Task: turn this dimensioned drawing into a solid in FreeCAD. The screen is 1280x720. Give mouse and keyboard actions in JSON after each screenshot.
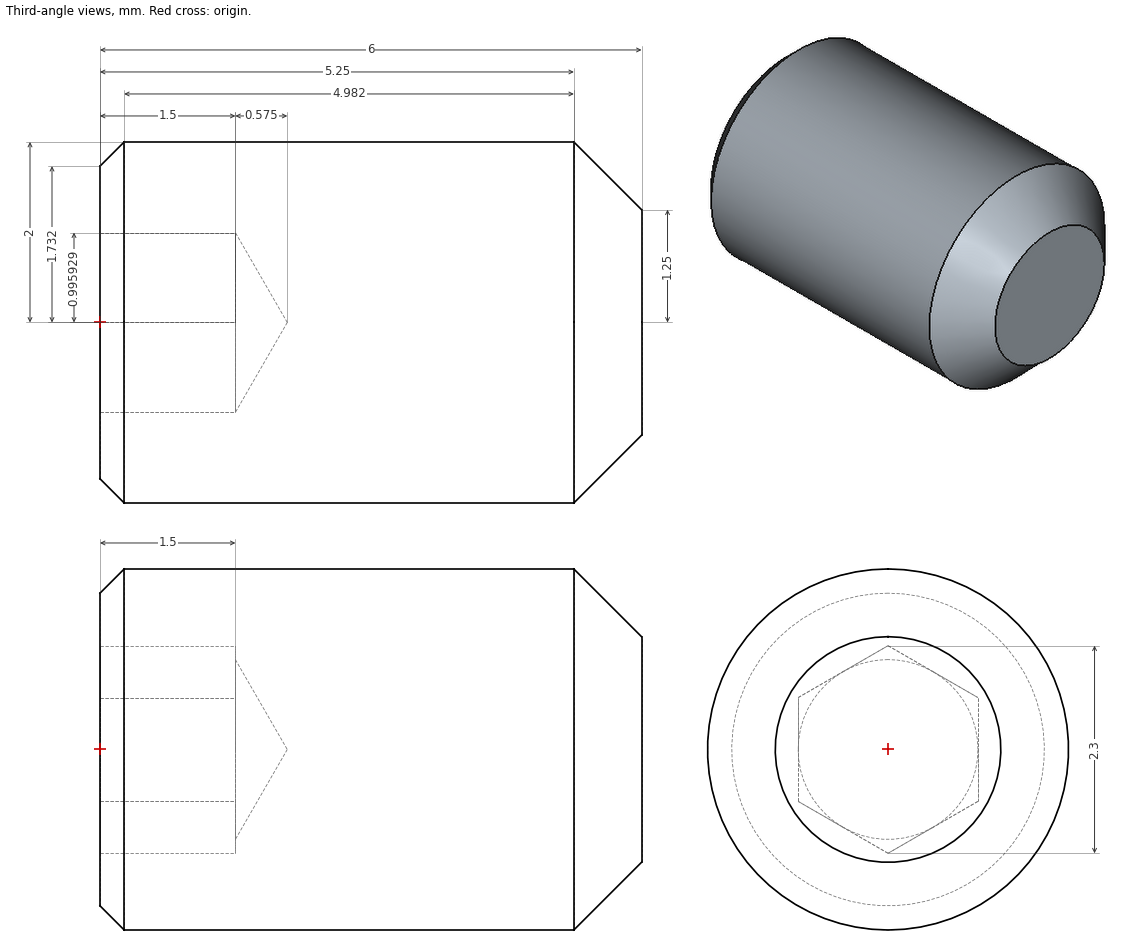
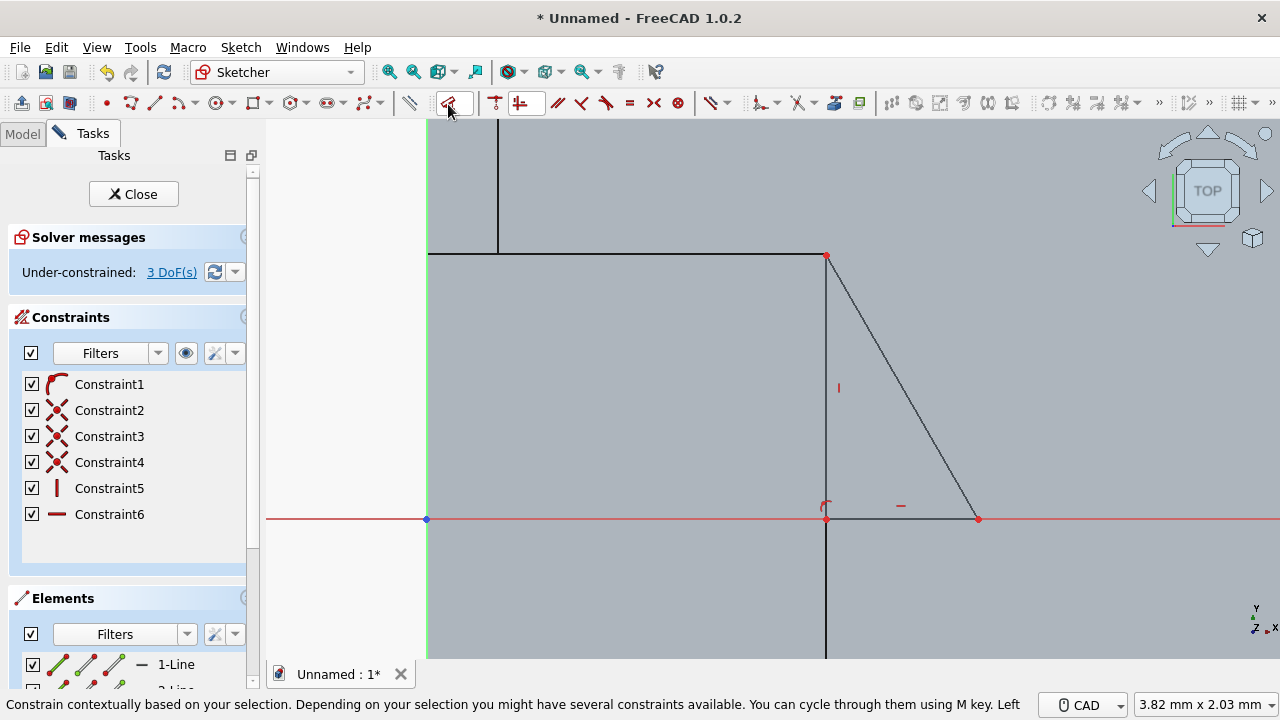
{"action": "left_click", "coordinate": [826, 519]}
{"action": "left_click", "coordinate": [626, 553]}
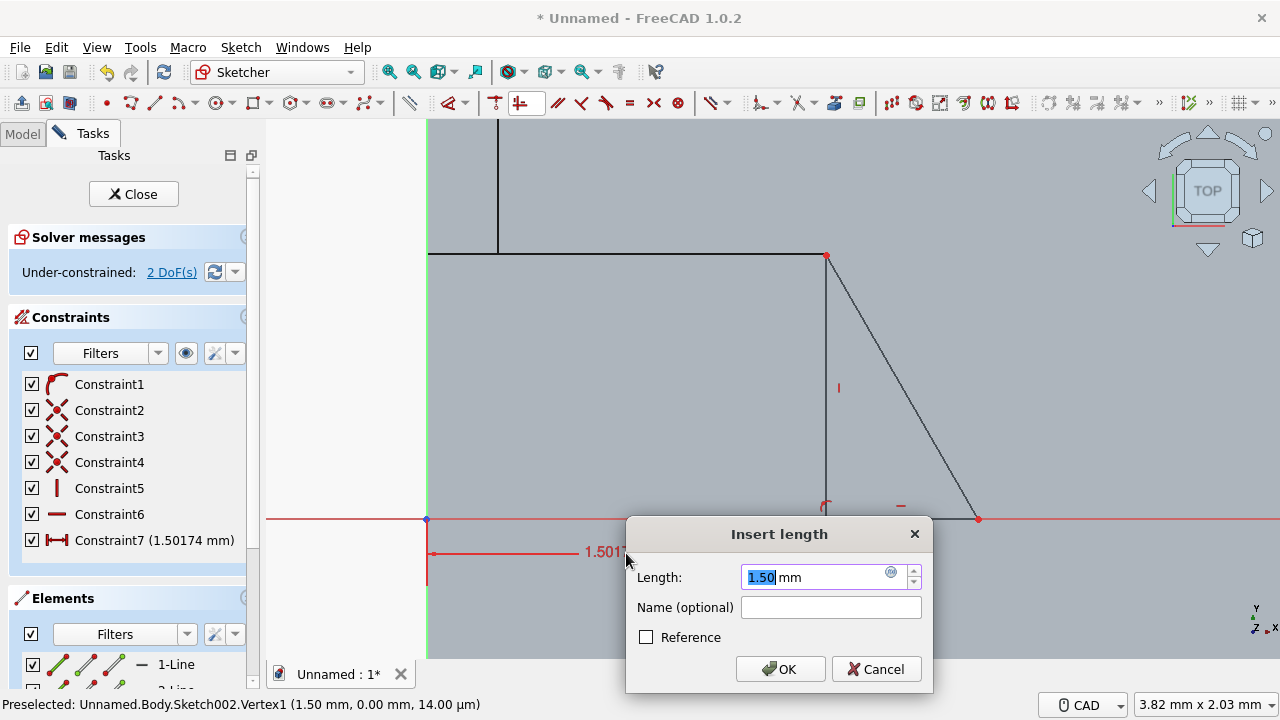
{"action": "type", "text": "1.5"}
{"action": "key", "text": "Return"}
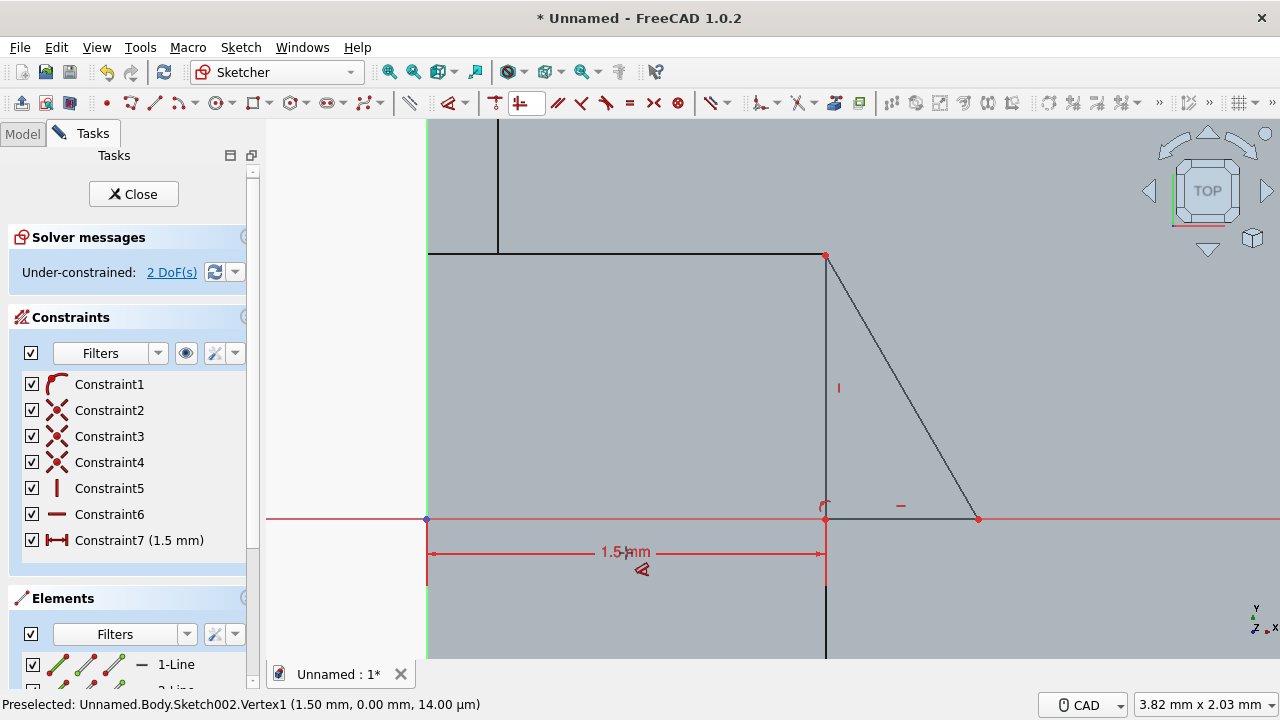
{"action": "left_click", "coordinate": [871, 519]}
{"action": "left_click", "coordinate": [902, 553]}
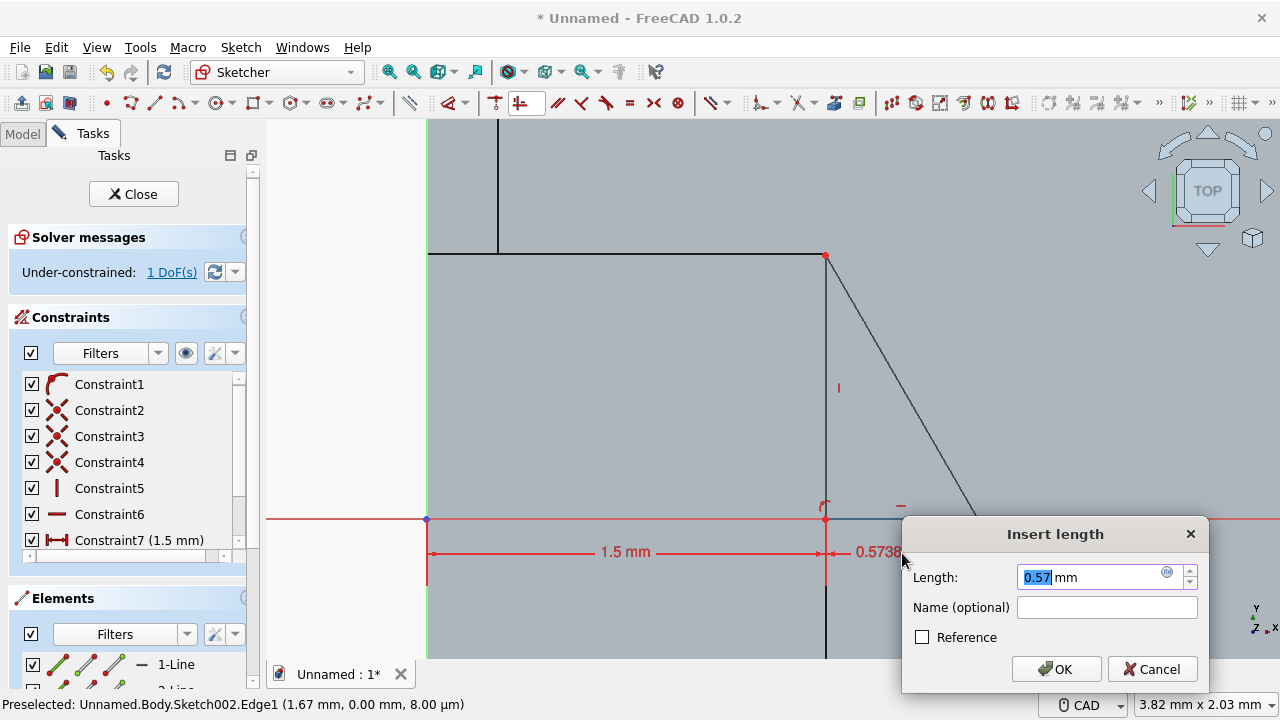
{"action": "type", "text": "0.575"}
{"action": "key", "text": "Return"}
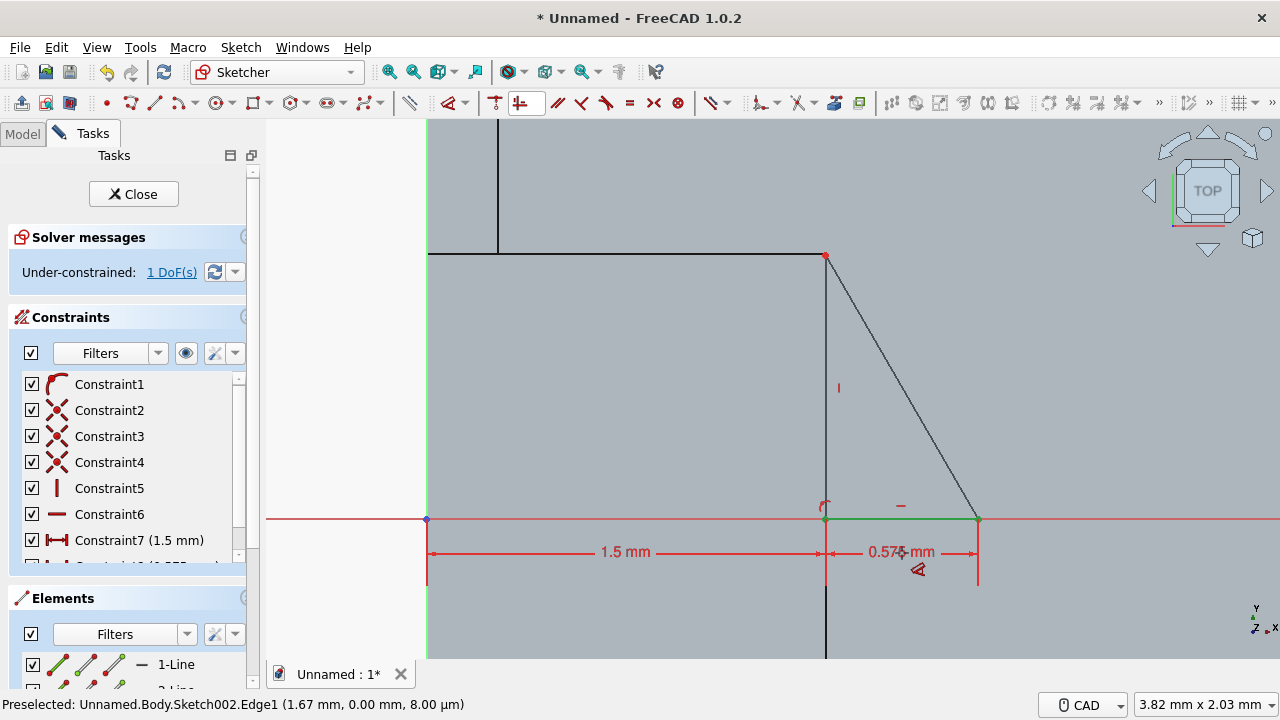
{"action": "left_click", "coordinate": [826, 334]}
{"action": "left_click", "coordinate": [860, 387]}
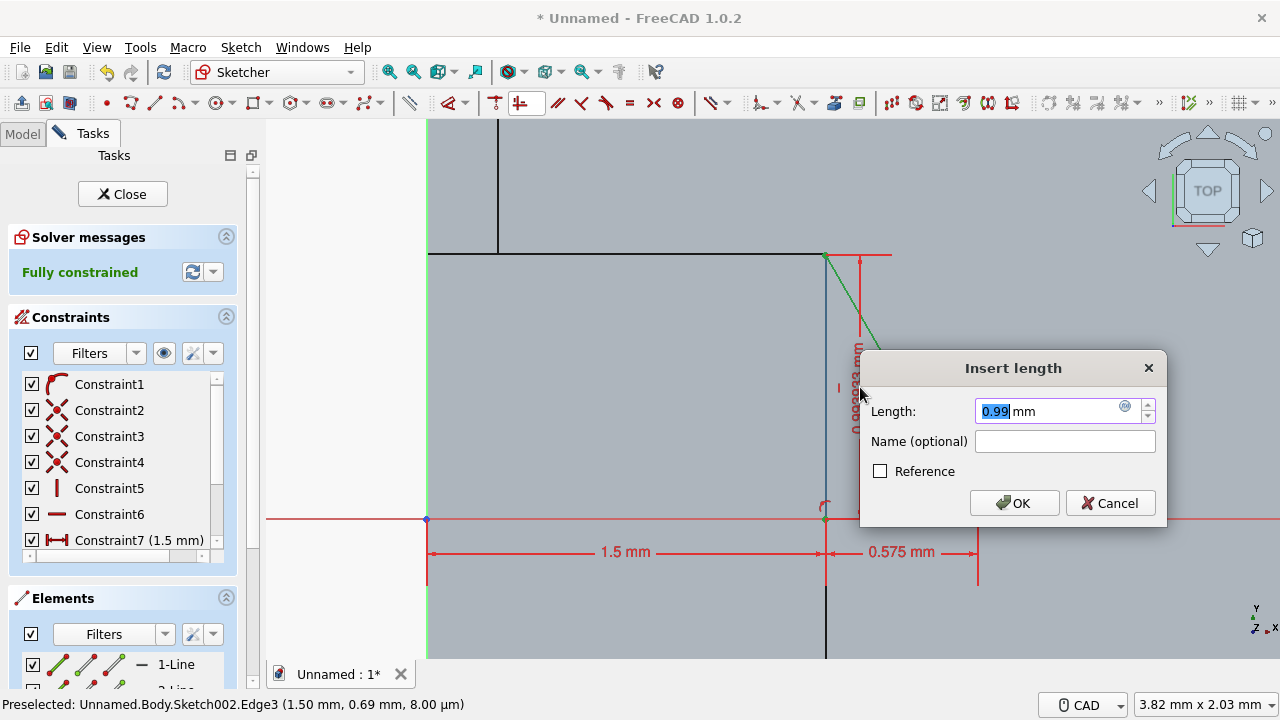
{"action": "type", "text": "0.995929"}
{"action": "key", "text": "Return"}
{"action": "key", "text": "Escape"}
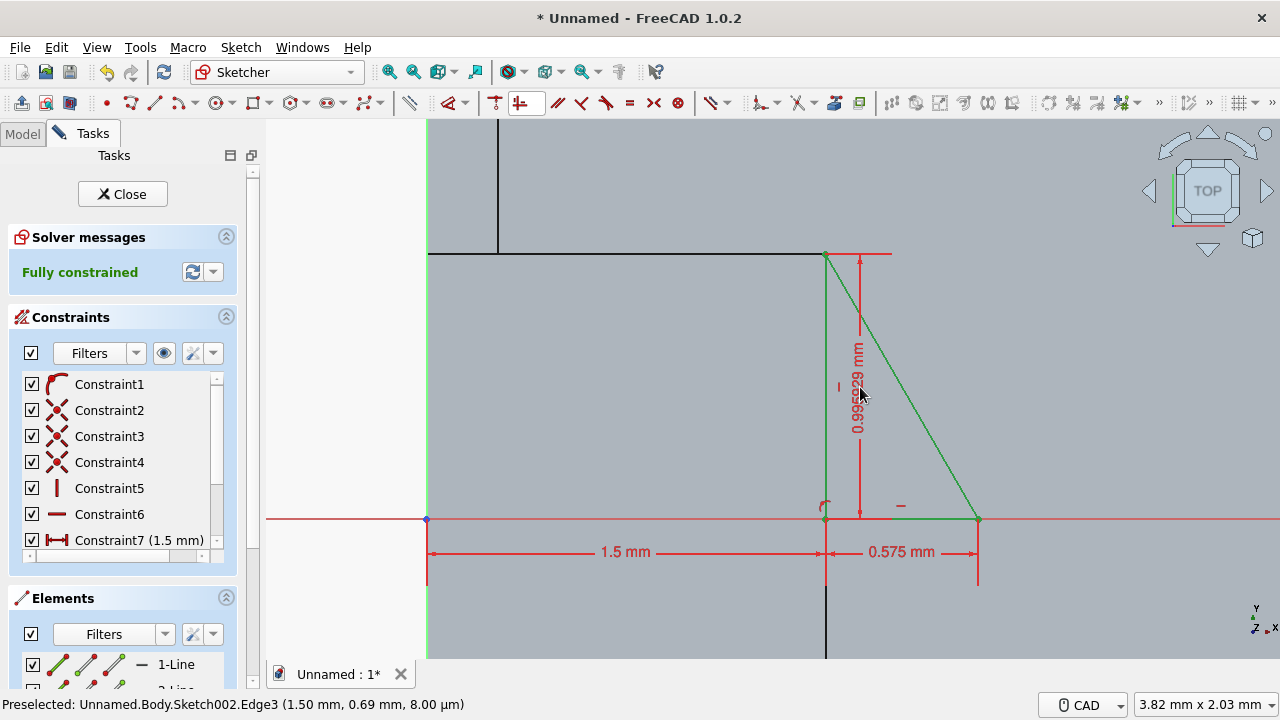
{"action": "left_click", "coordinate": [123, 194]}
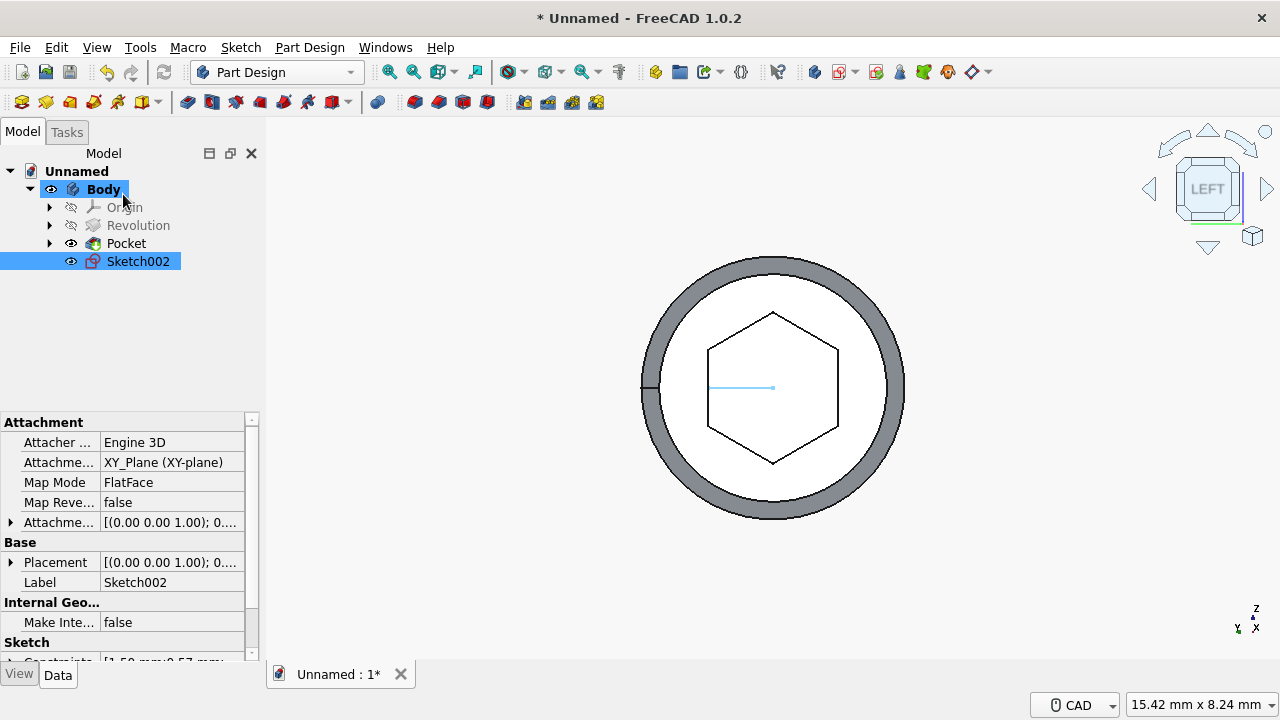
{"action": "left_click", "coordinate": [236, 102]}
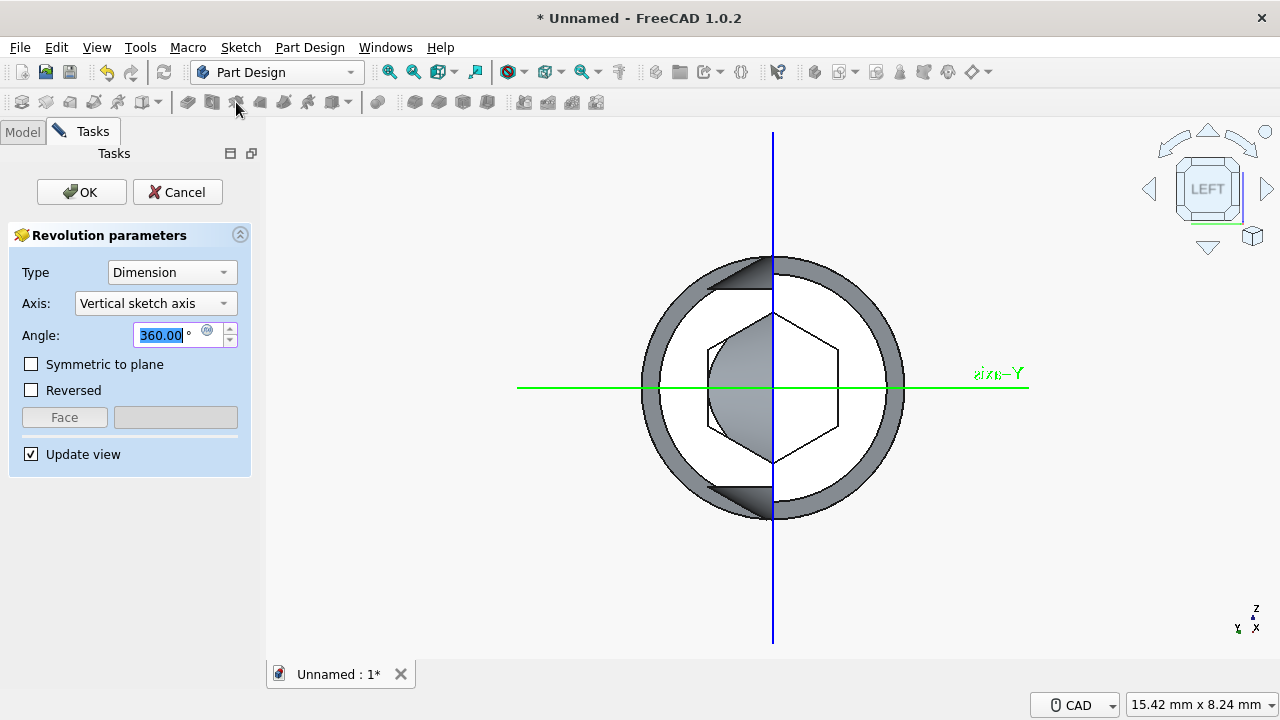
{"action": "left_click", "coordinate": [156, 304]}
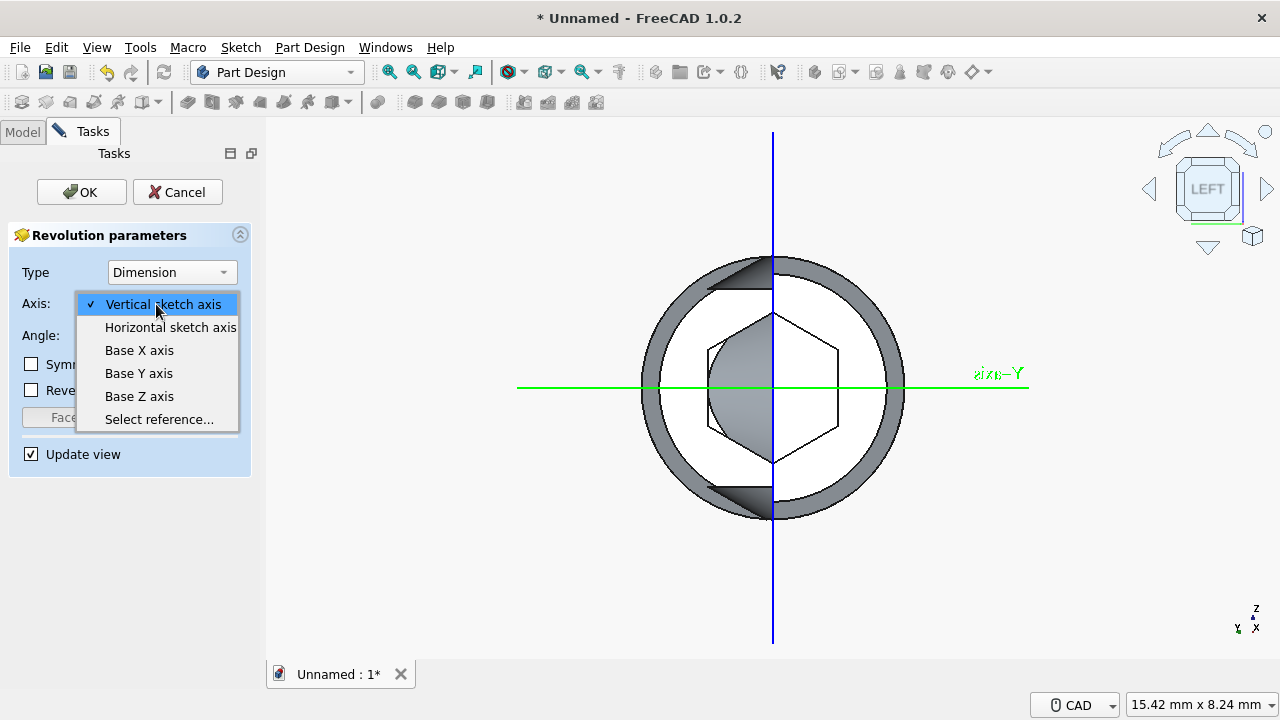
{"action": "left_click", "coordinate": [156, 328]}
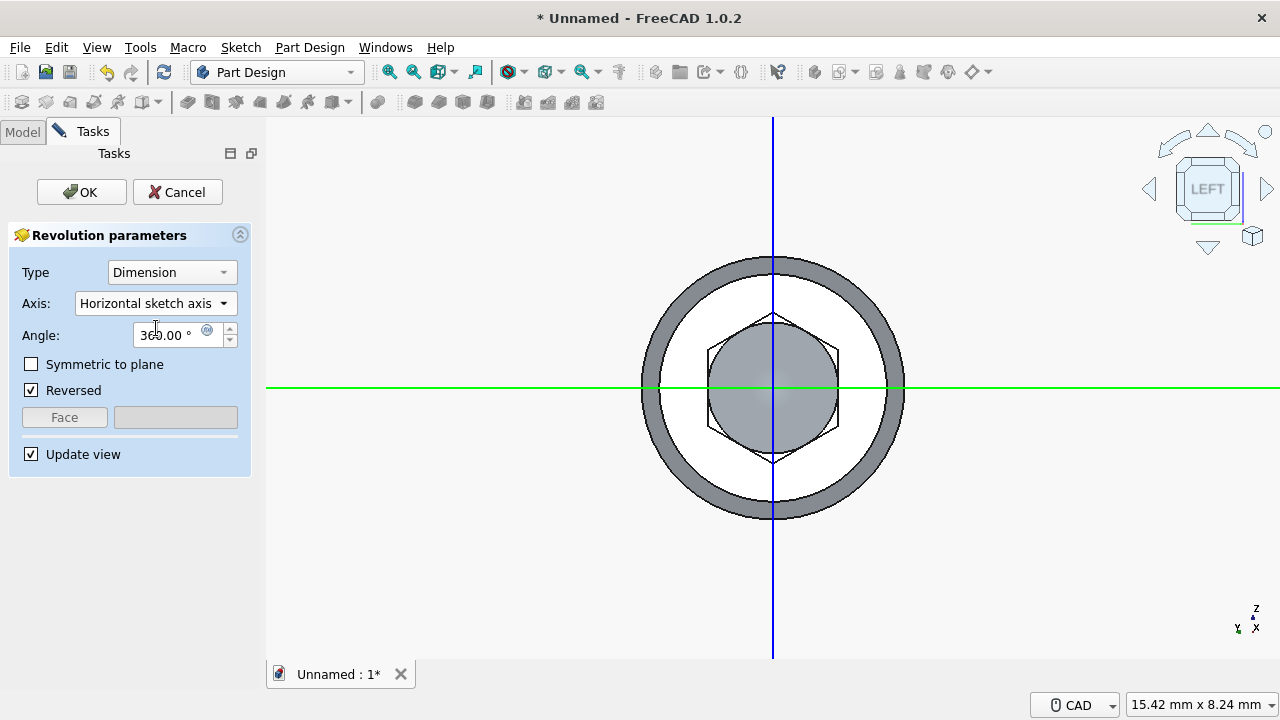
{"action": "left_click", "coordinate": [82, 192]}